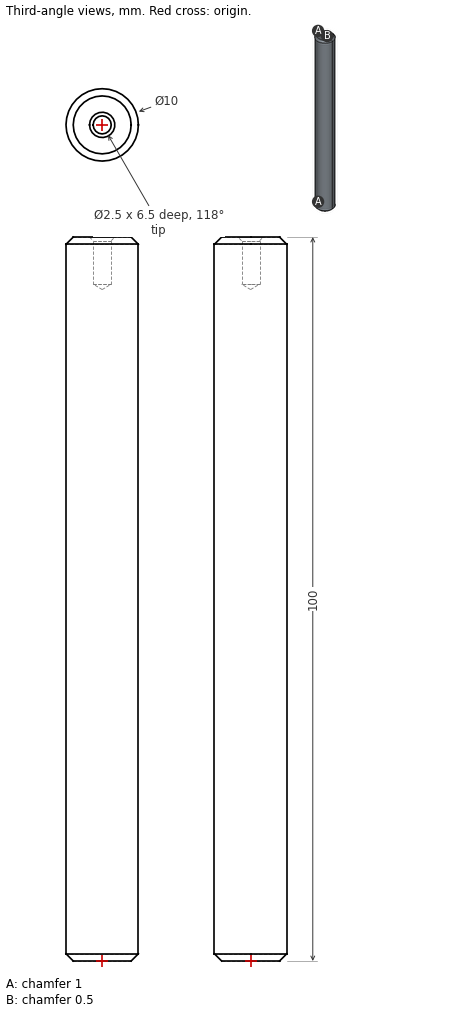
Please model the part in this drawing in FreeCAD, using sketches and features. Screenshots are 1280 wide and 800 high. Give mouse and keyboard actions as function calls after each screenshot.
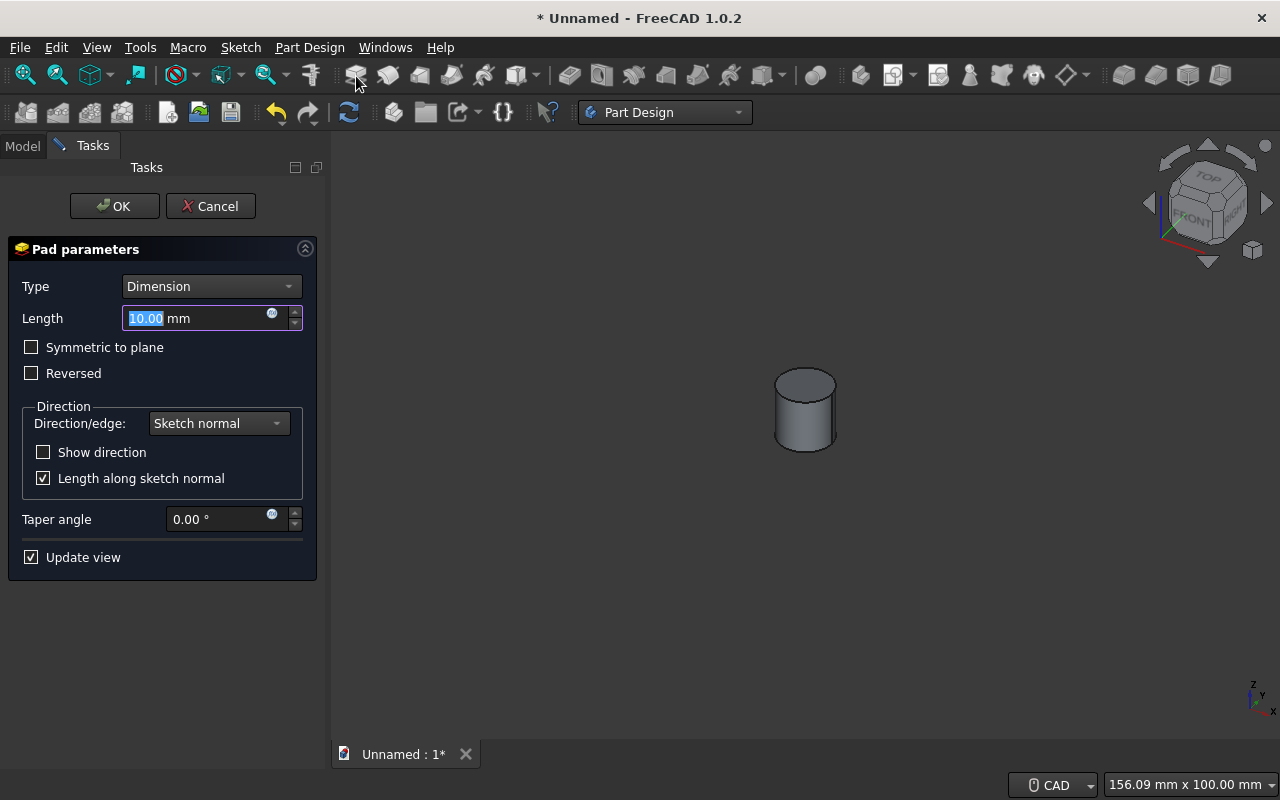
text(100)
key(Tab)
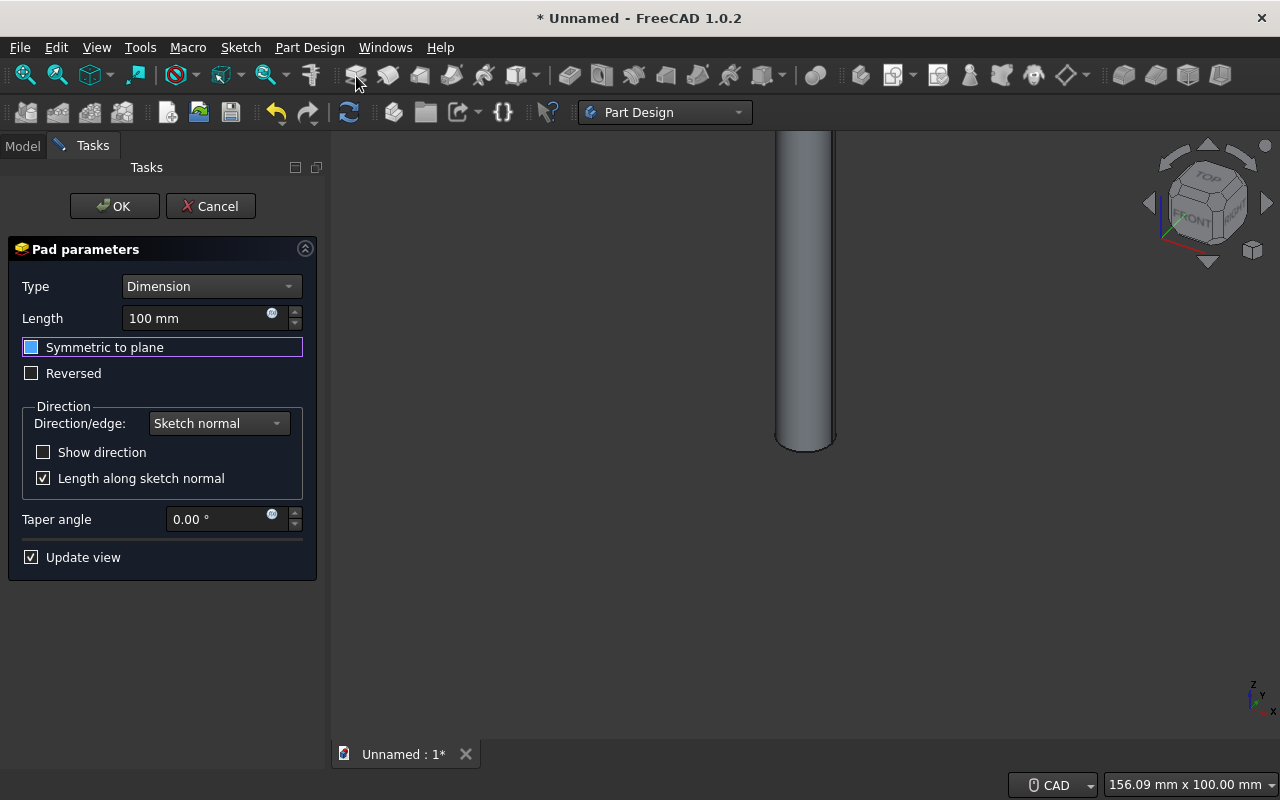
click(115, 206)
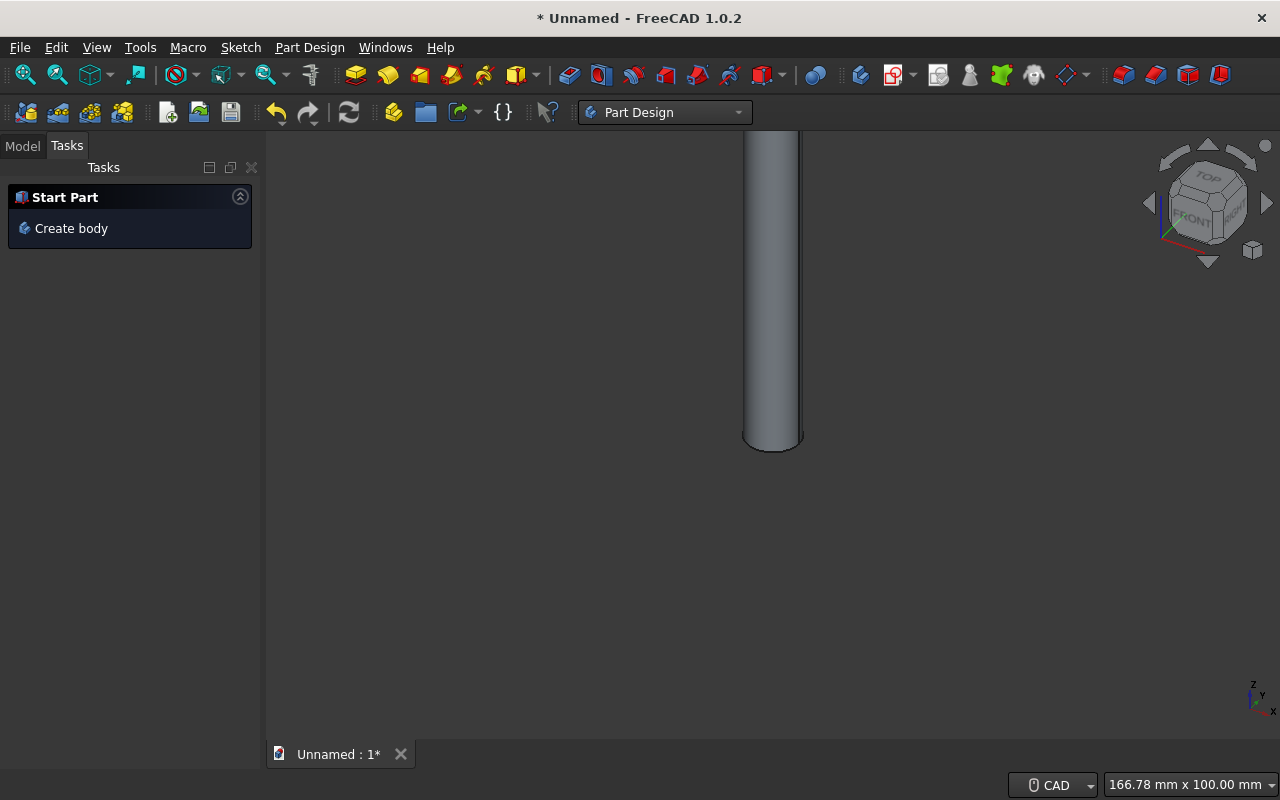
click(26, 76)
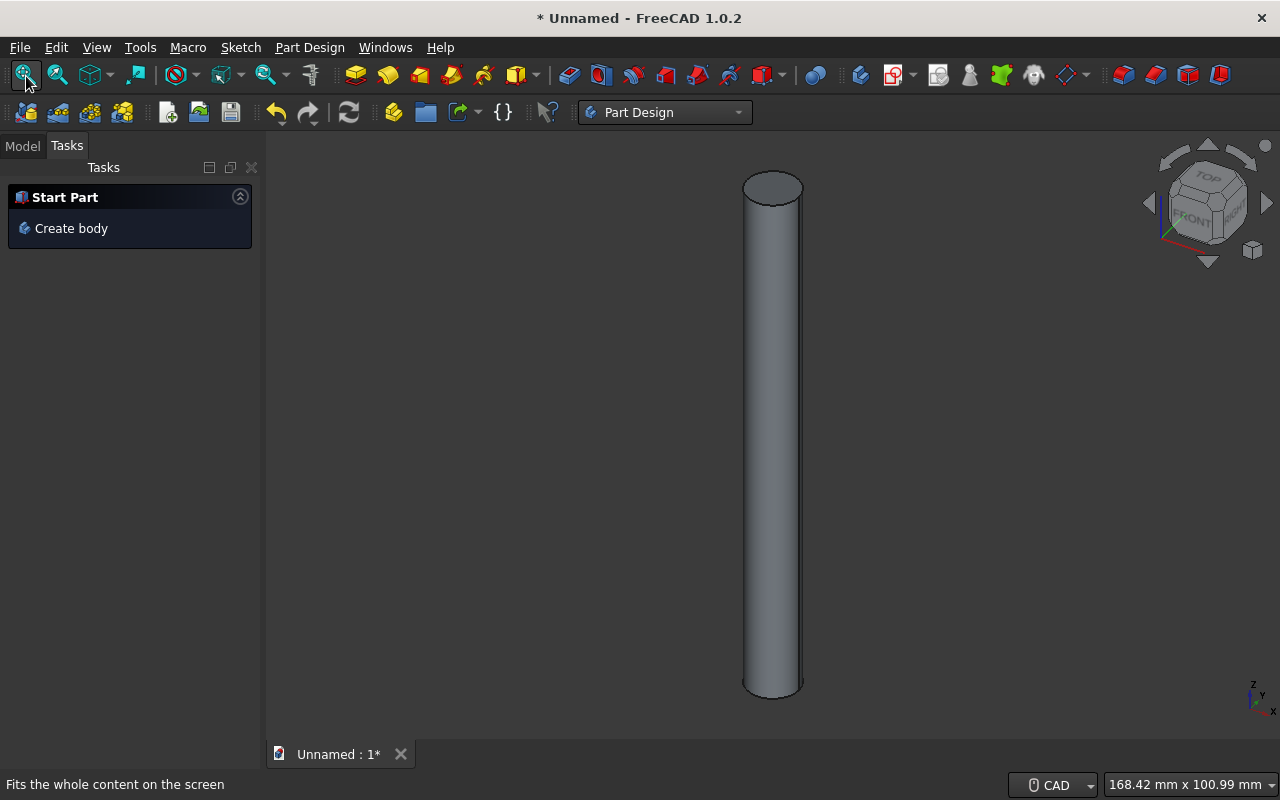
click(773, 187)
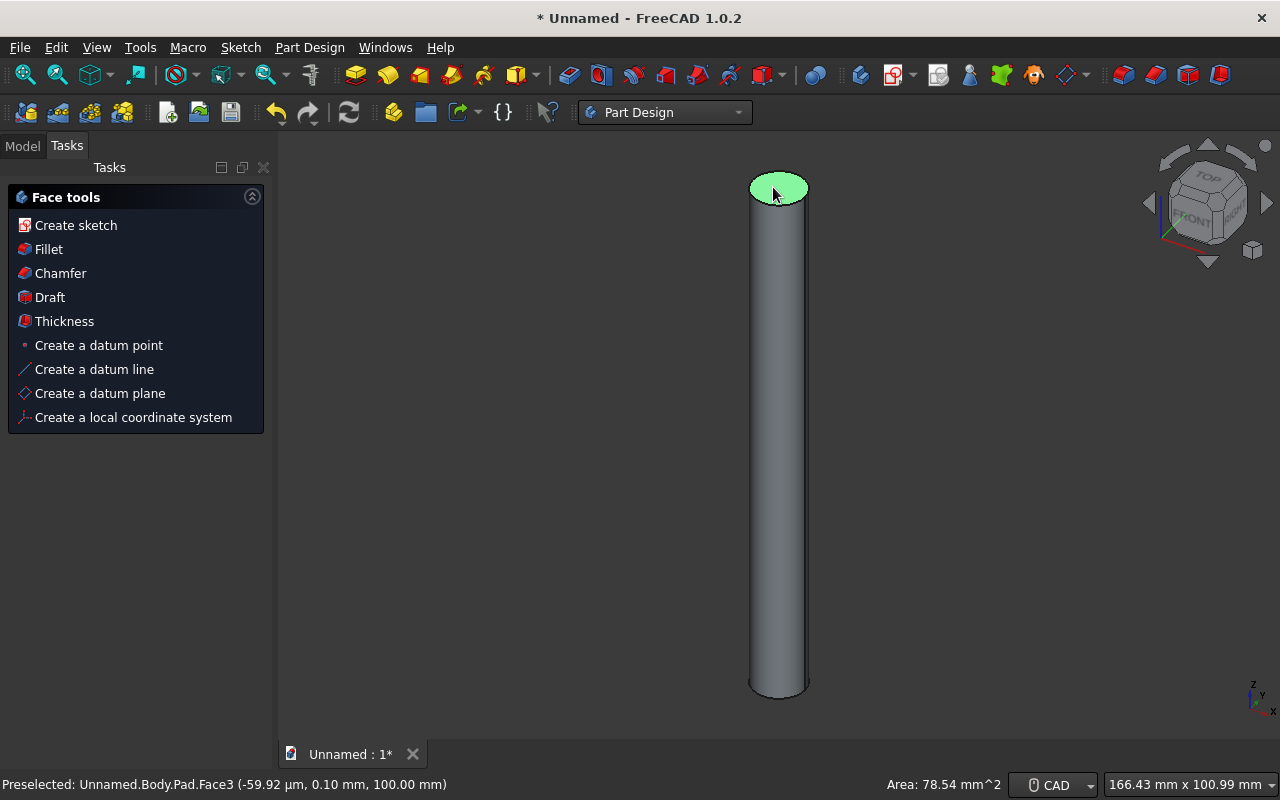
click(894, 76)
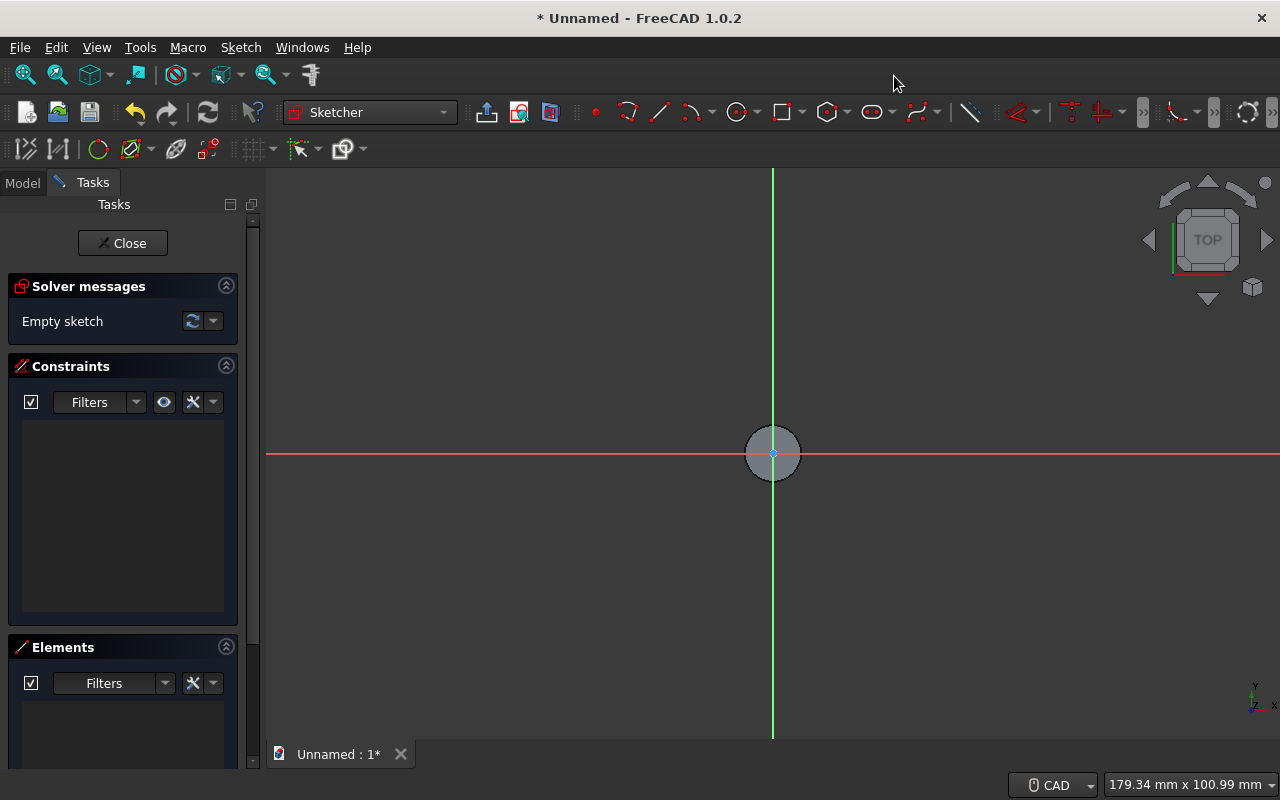
scroll(777, 454, up, 15)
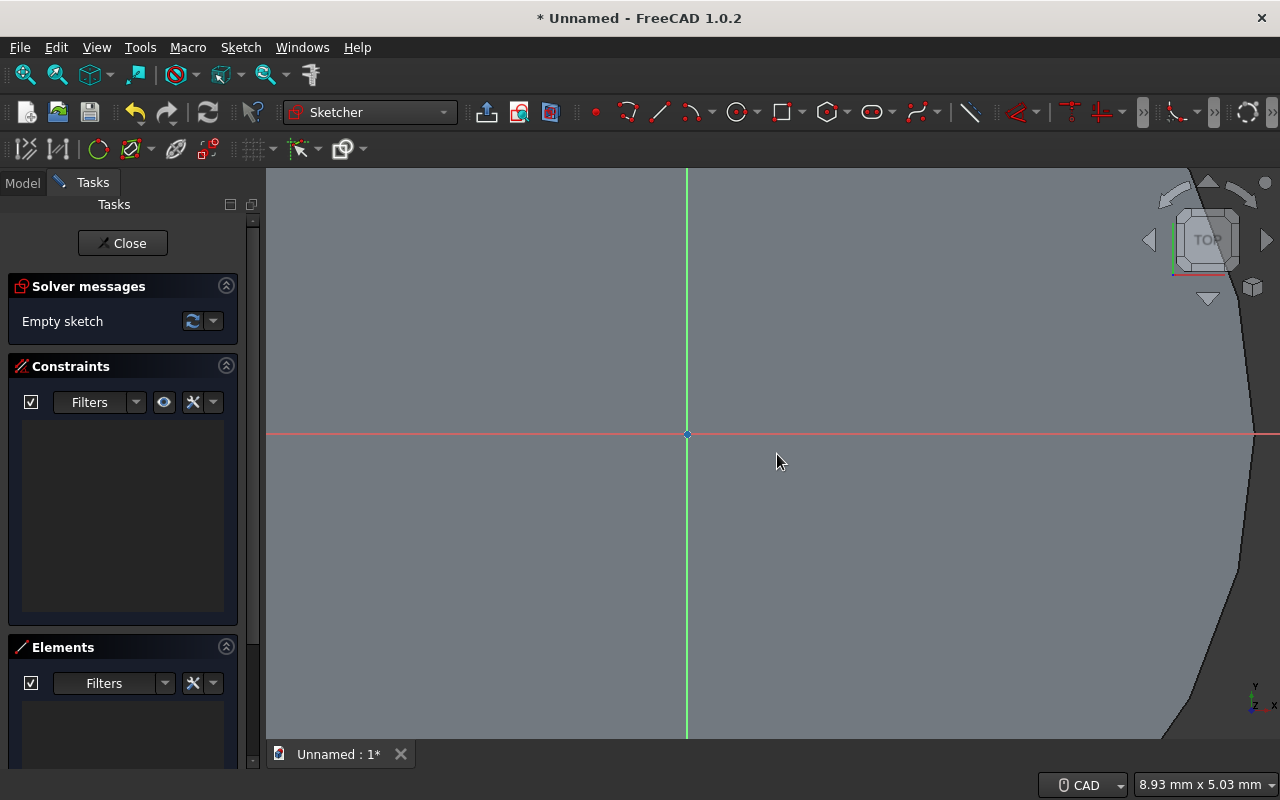
key(g)
key(c)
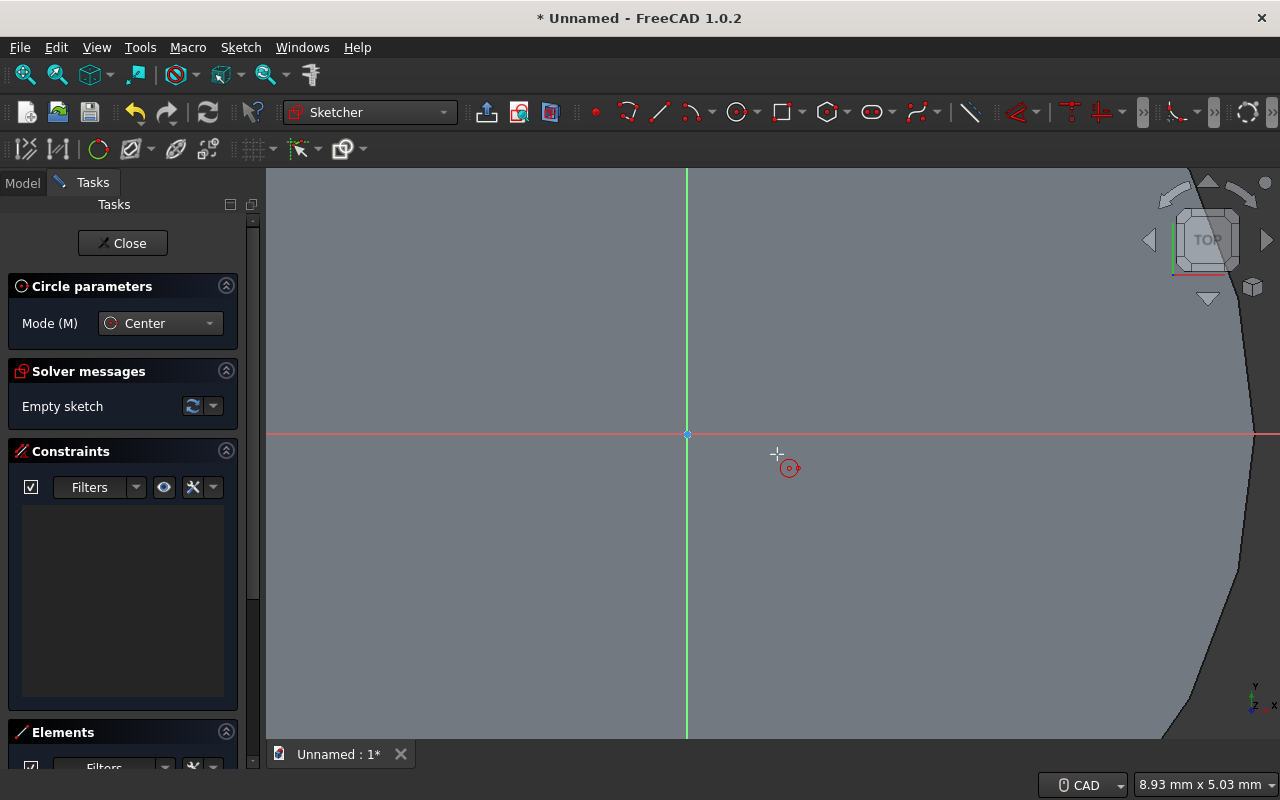
click(687, 434)
move(787, 334)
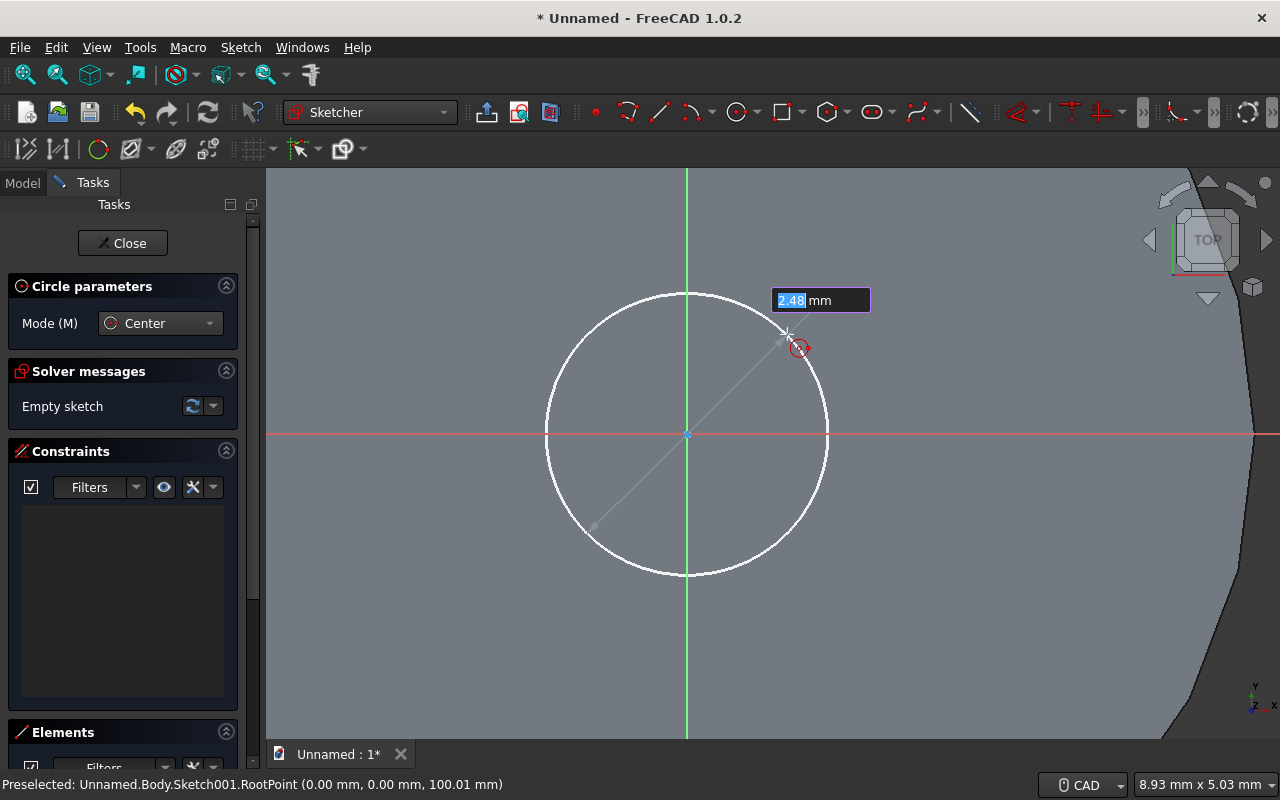
text(2.5)
key(Return)
key(Escape)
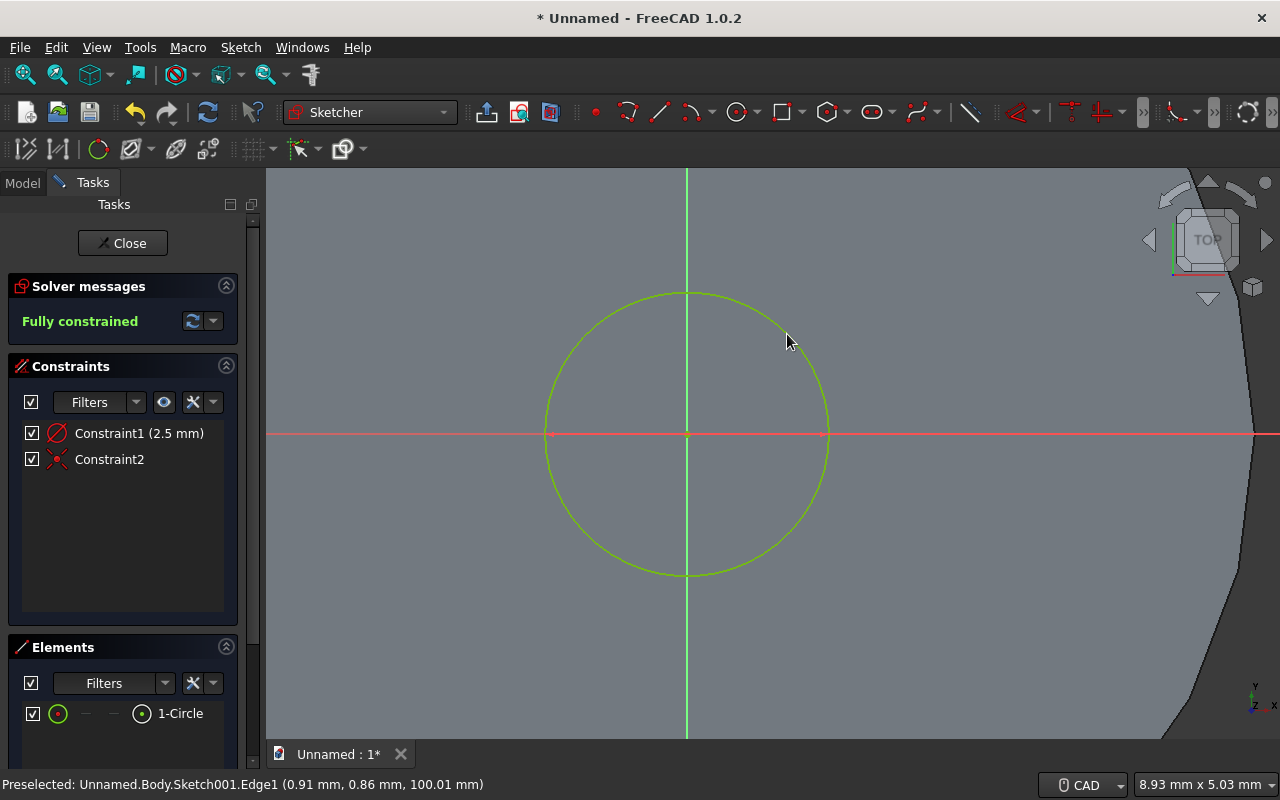
click(123, 243)